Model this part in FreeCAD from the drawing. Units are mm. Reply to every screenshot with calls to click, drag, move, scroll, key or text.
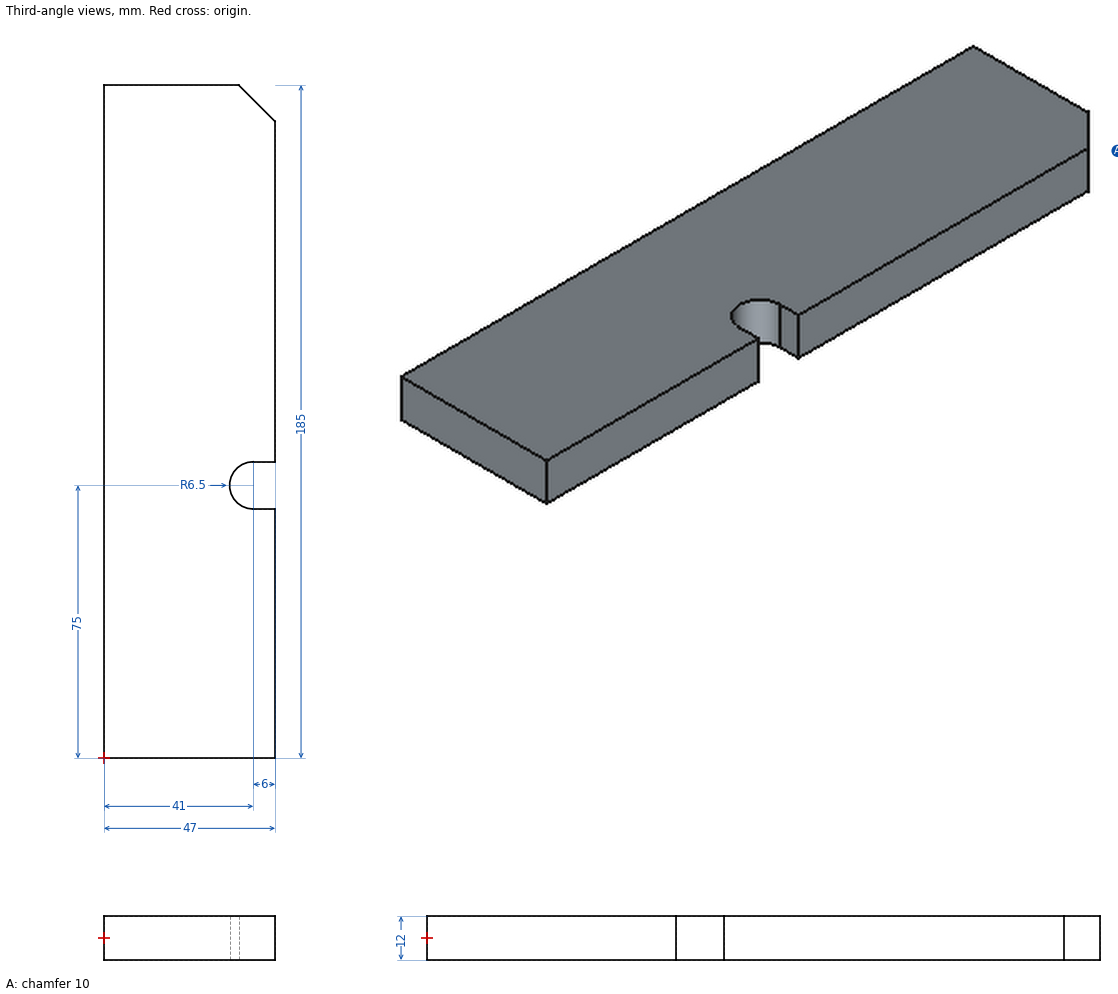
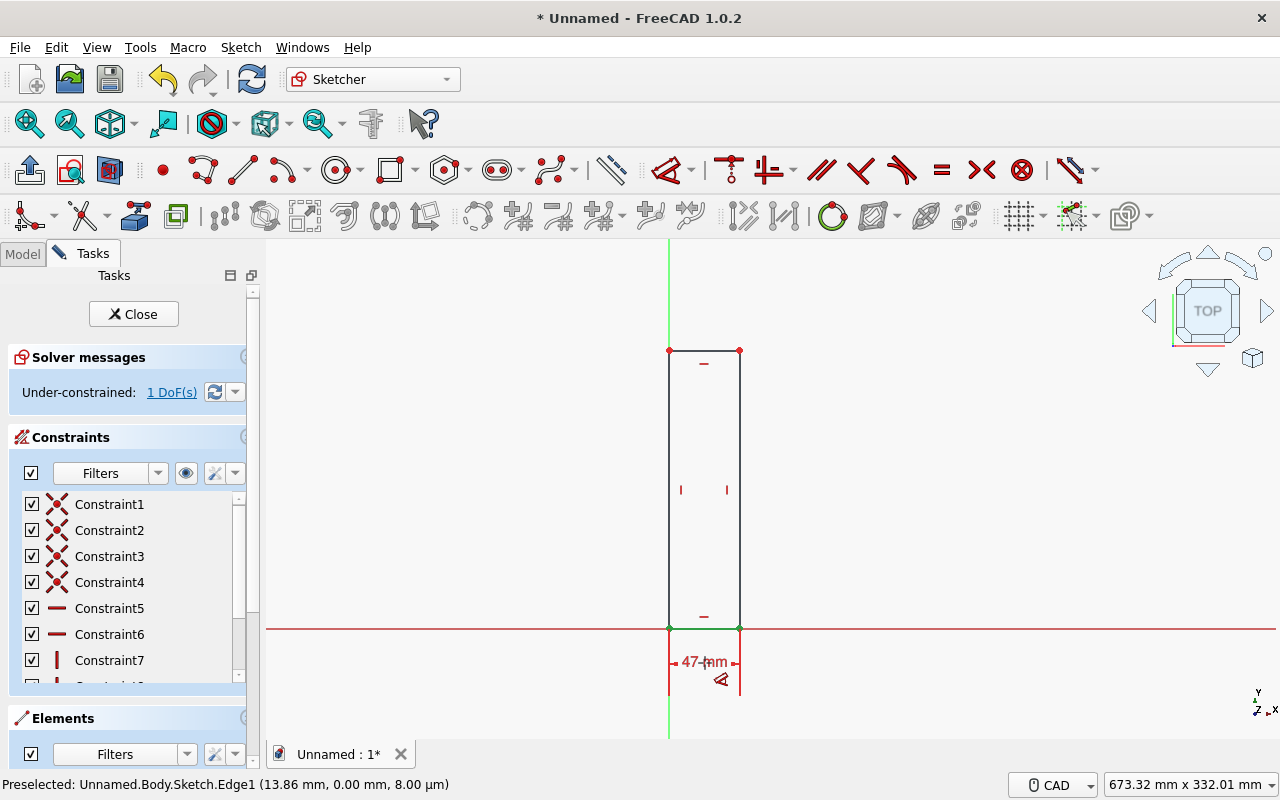
click(740, 545)
click(774, 490)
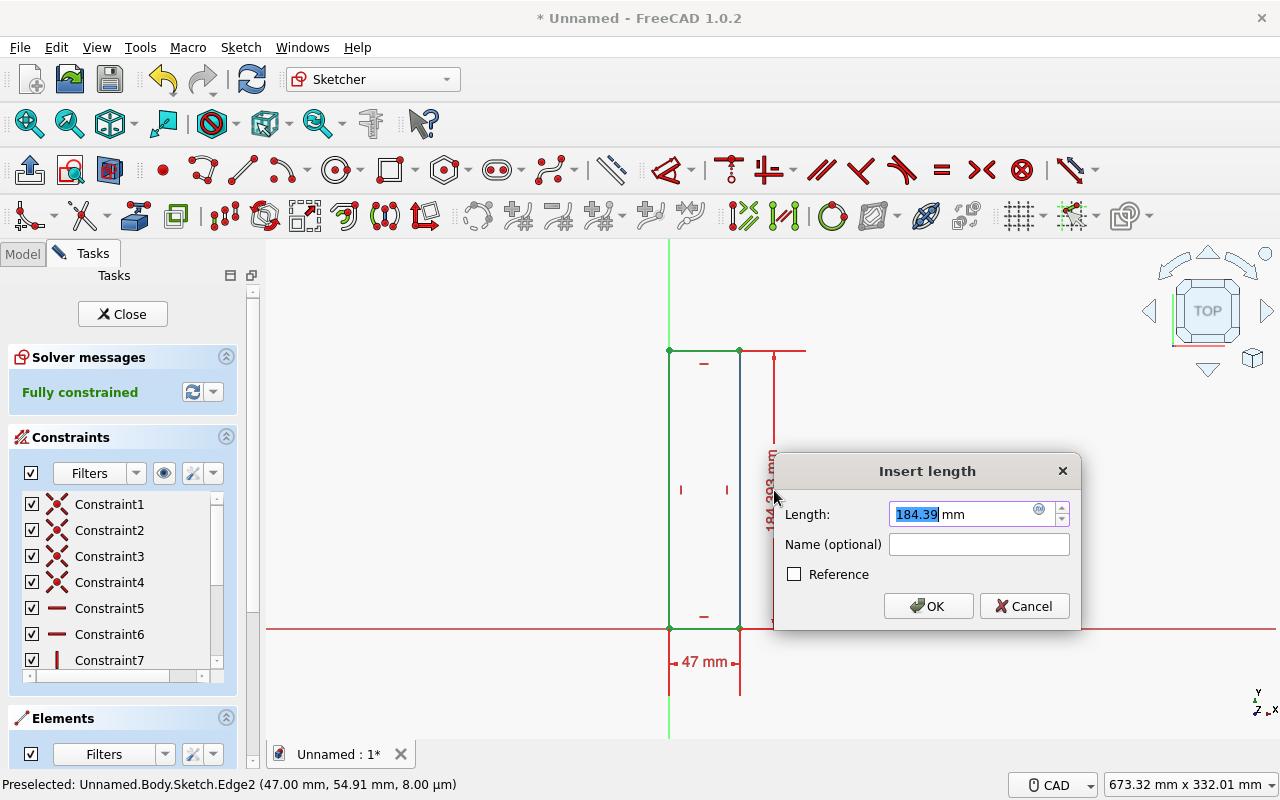
text(185)
key(Return)
key(Escape)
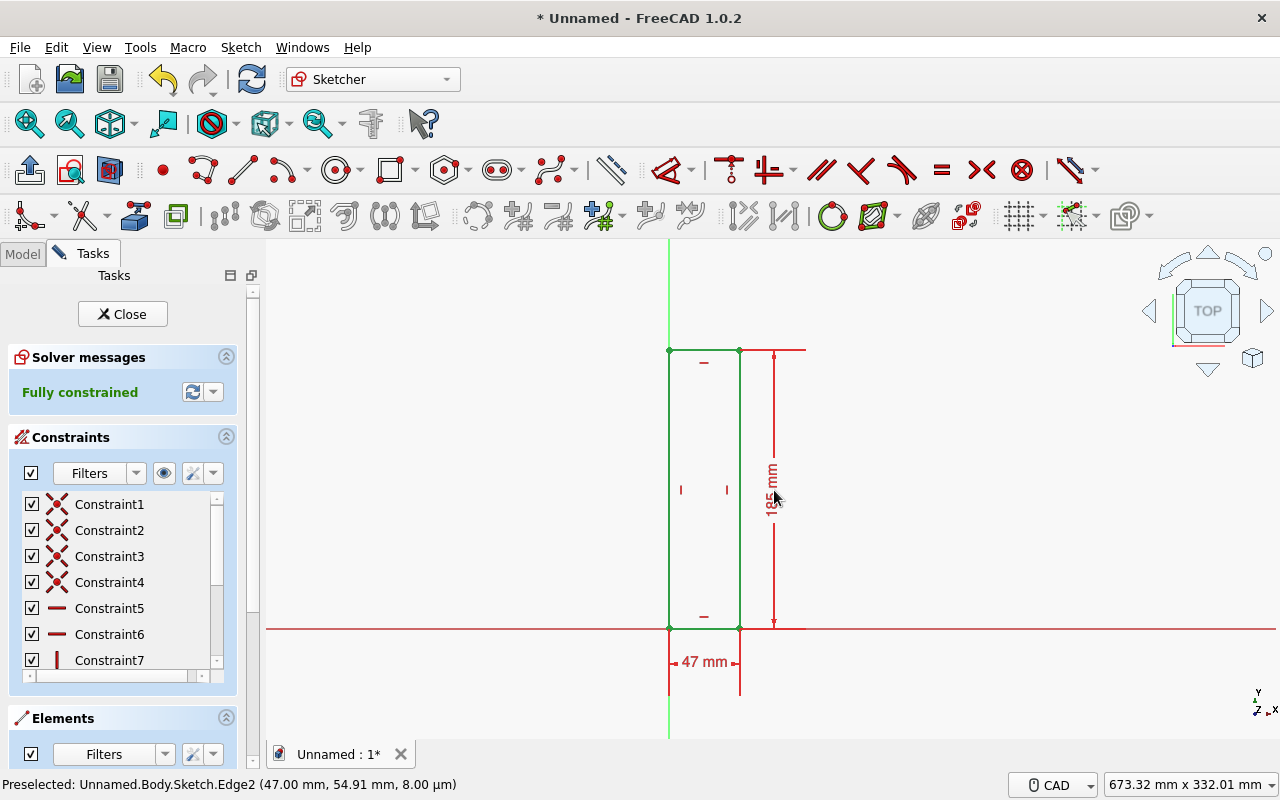
click(123, 314)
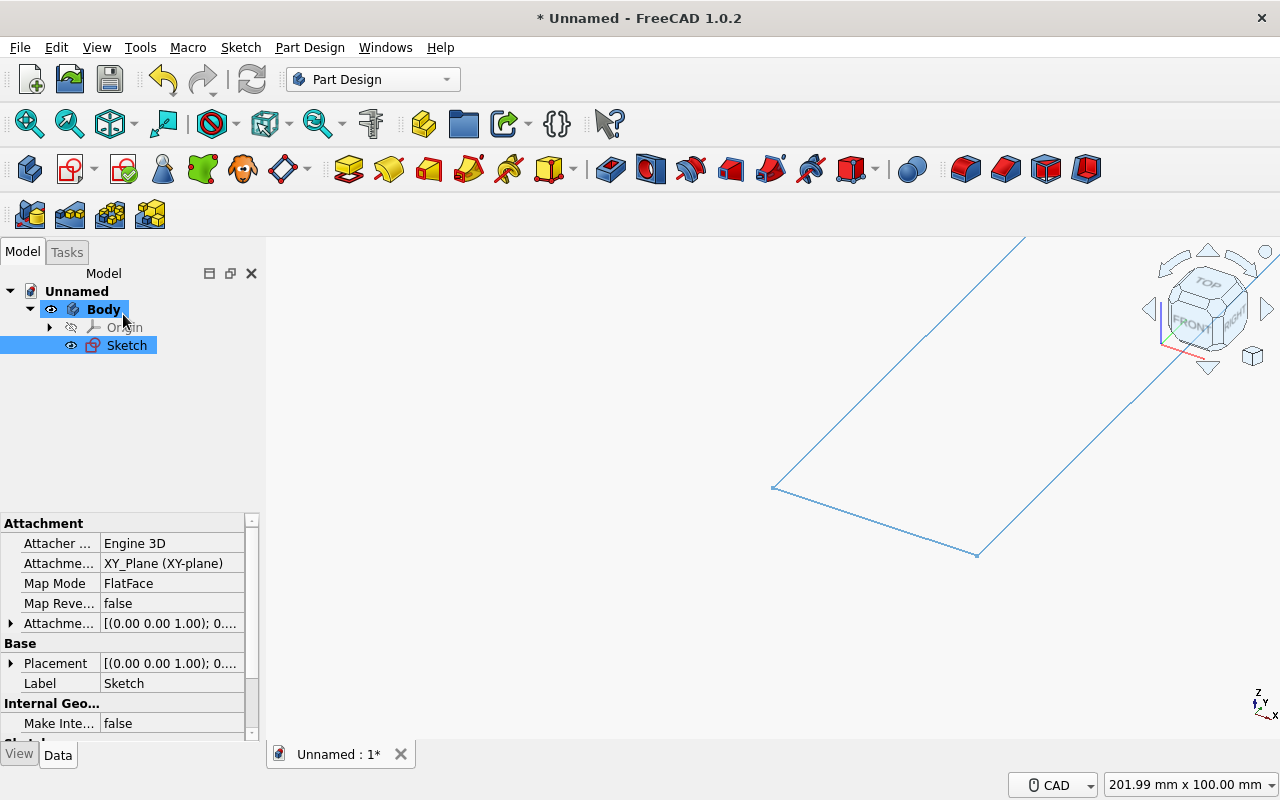
click(350, 170)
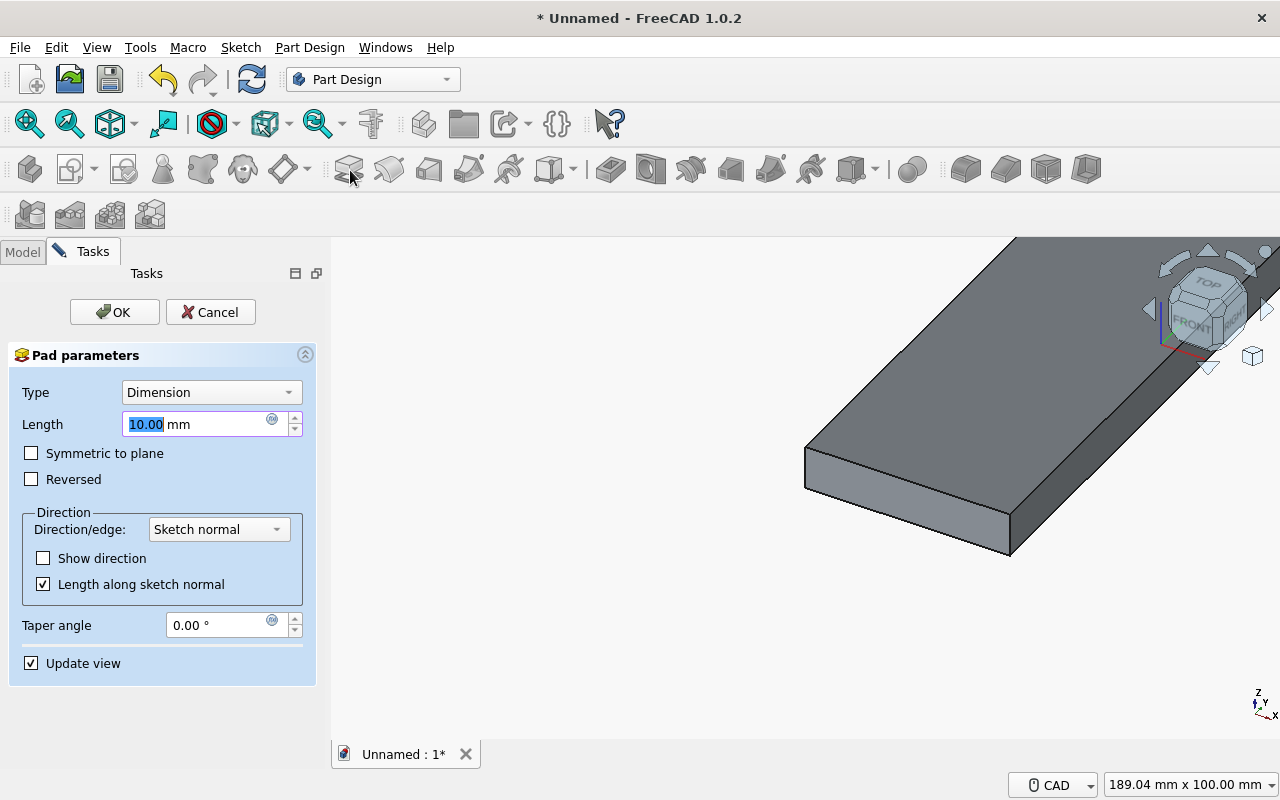
text(12)
key(Tab)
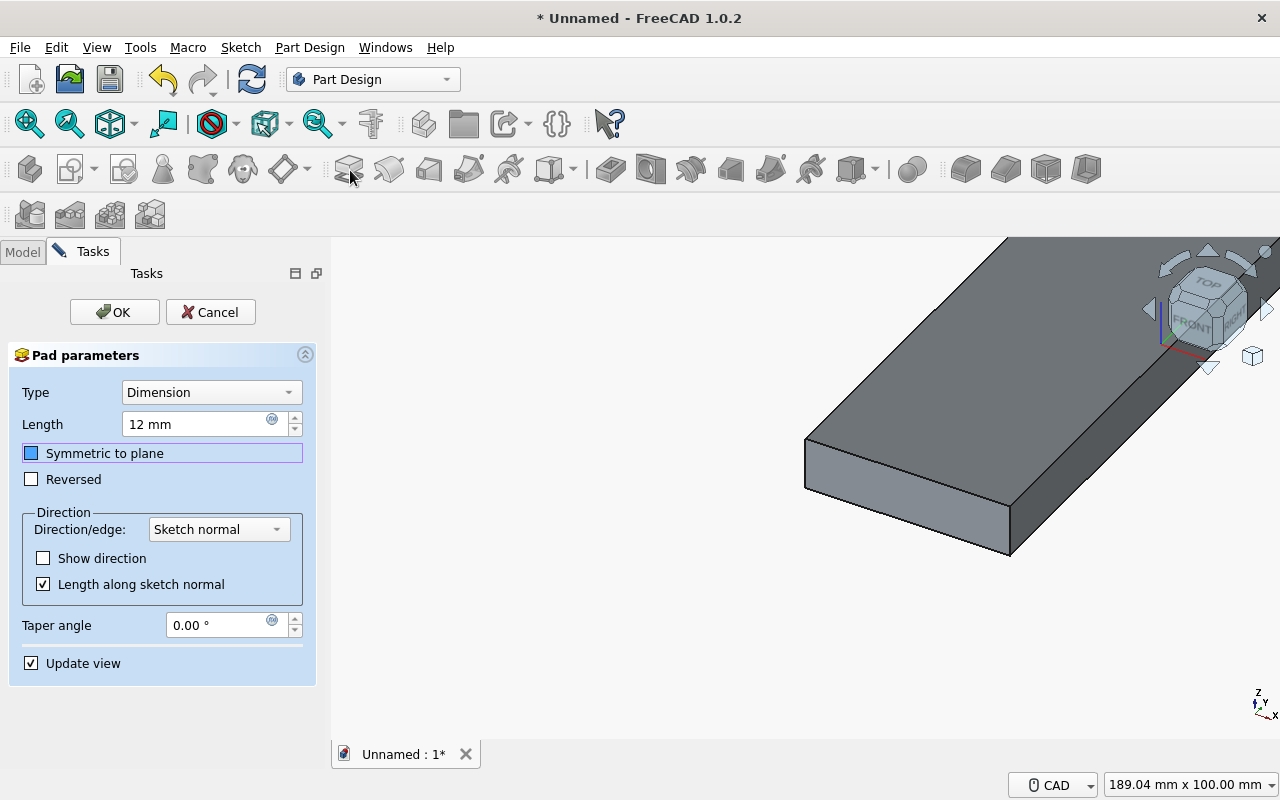
click(30, 453)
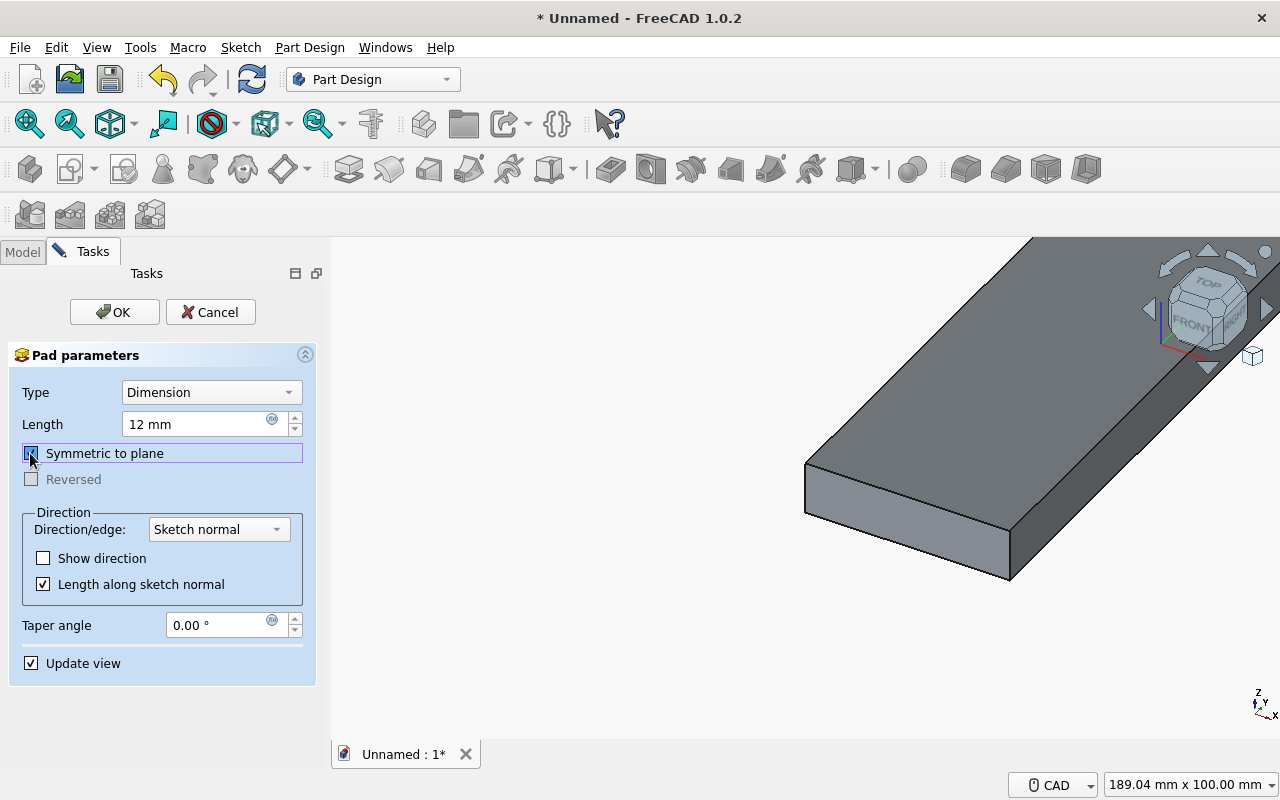
click(115, 312)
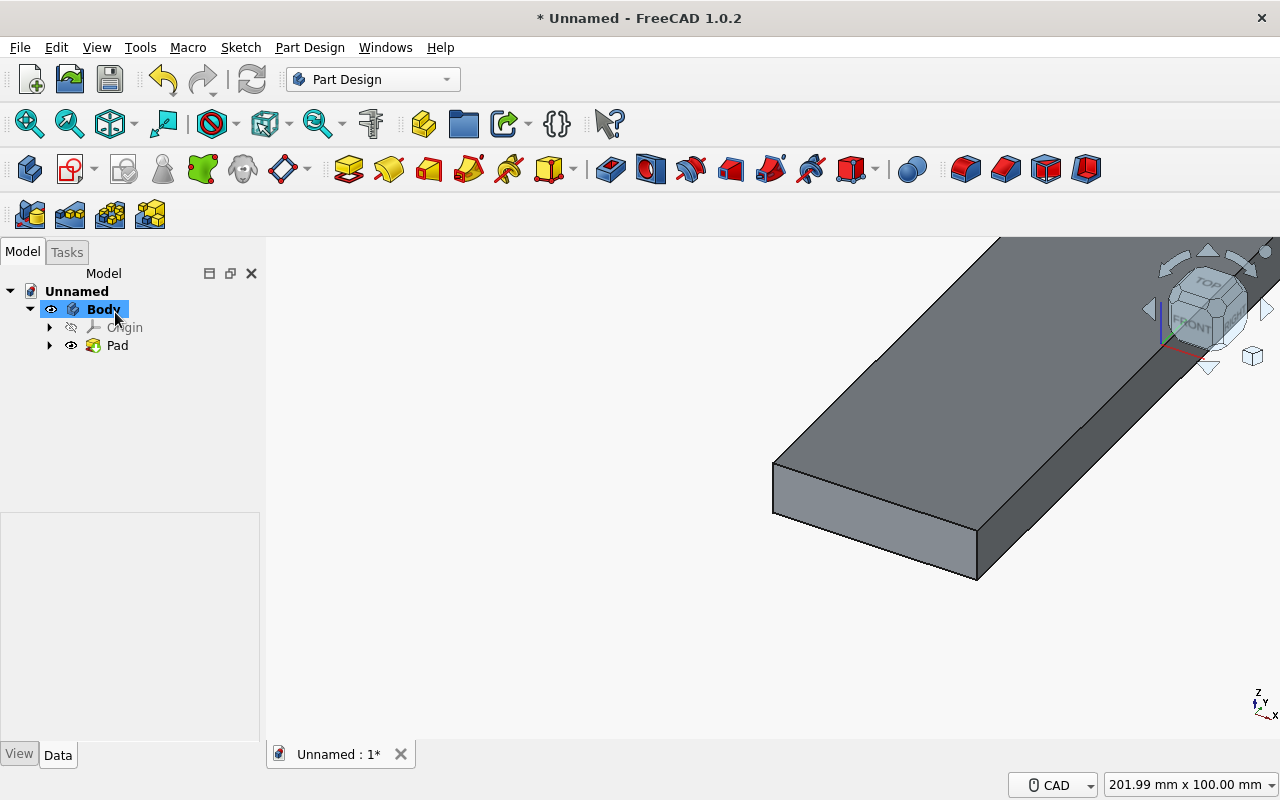
click(30, 124)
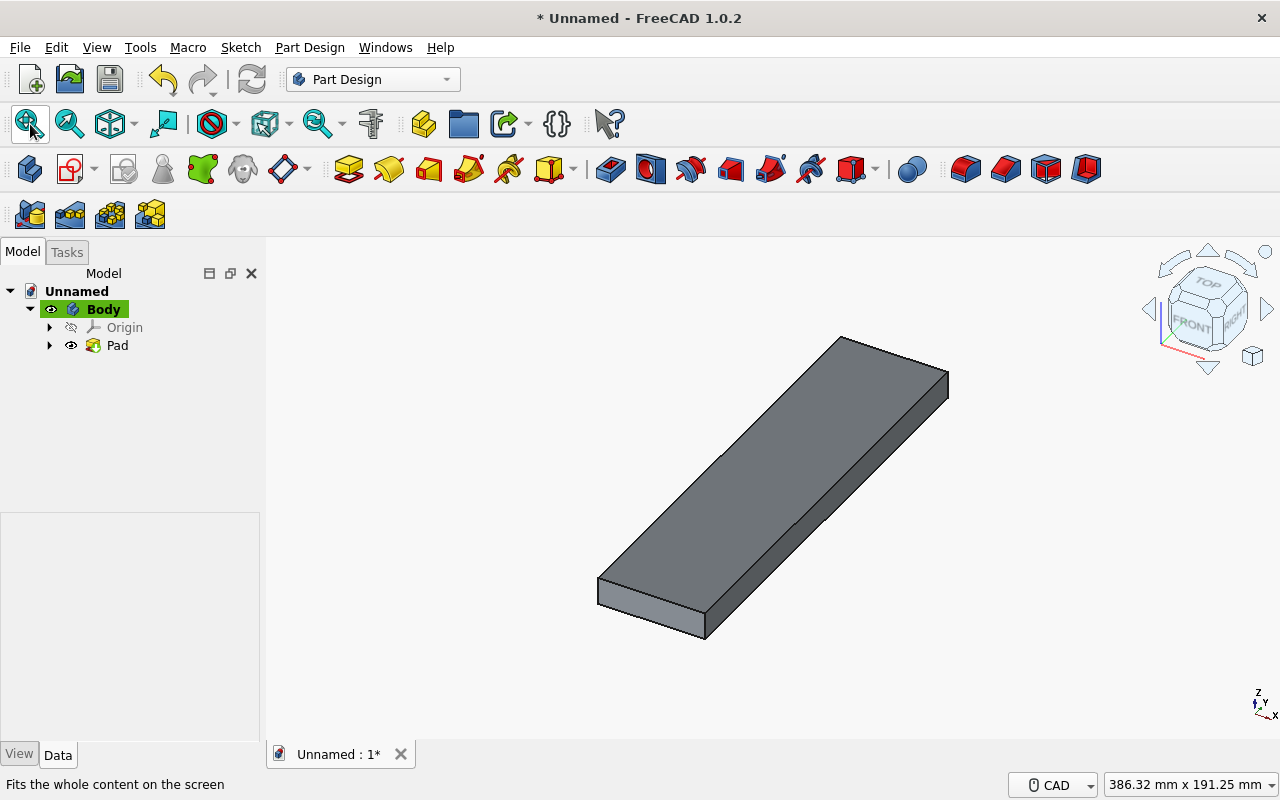
key(0)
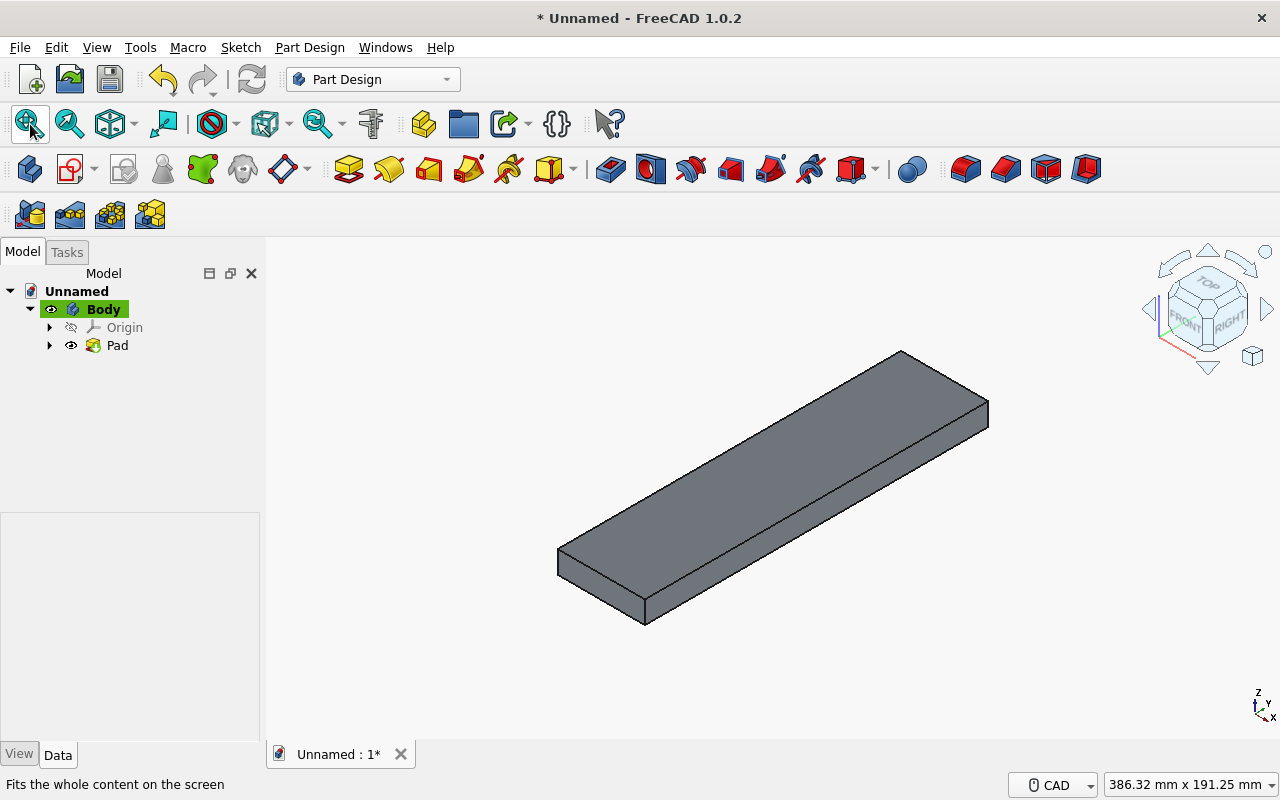
key(2)